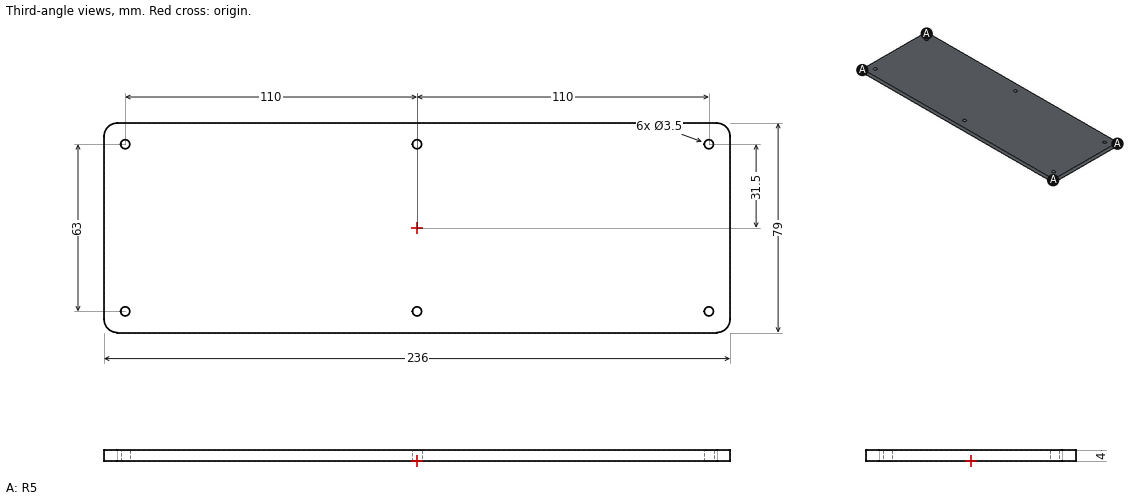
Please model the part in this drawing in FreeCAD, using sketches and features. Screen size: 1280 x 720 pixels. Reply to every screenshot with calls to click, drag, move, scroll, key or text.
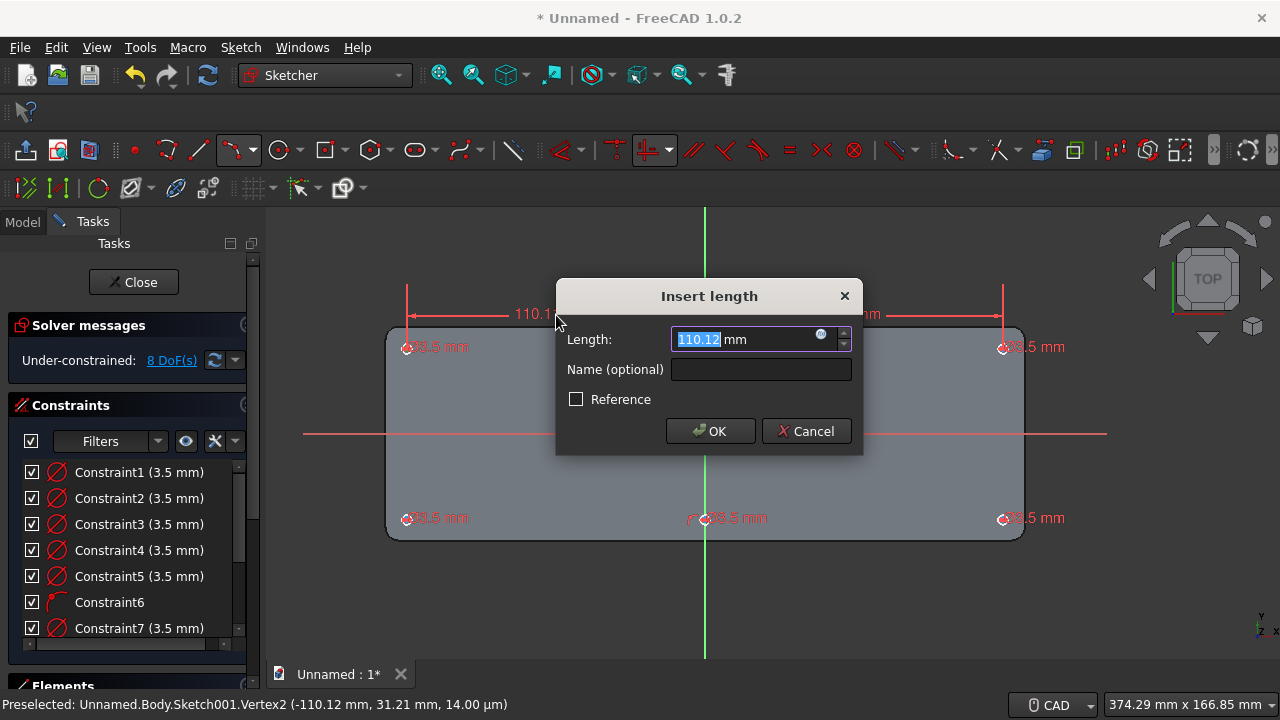
text(110)
key(Return)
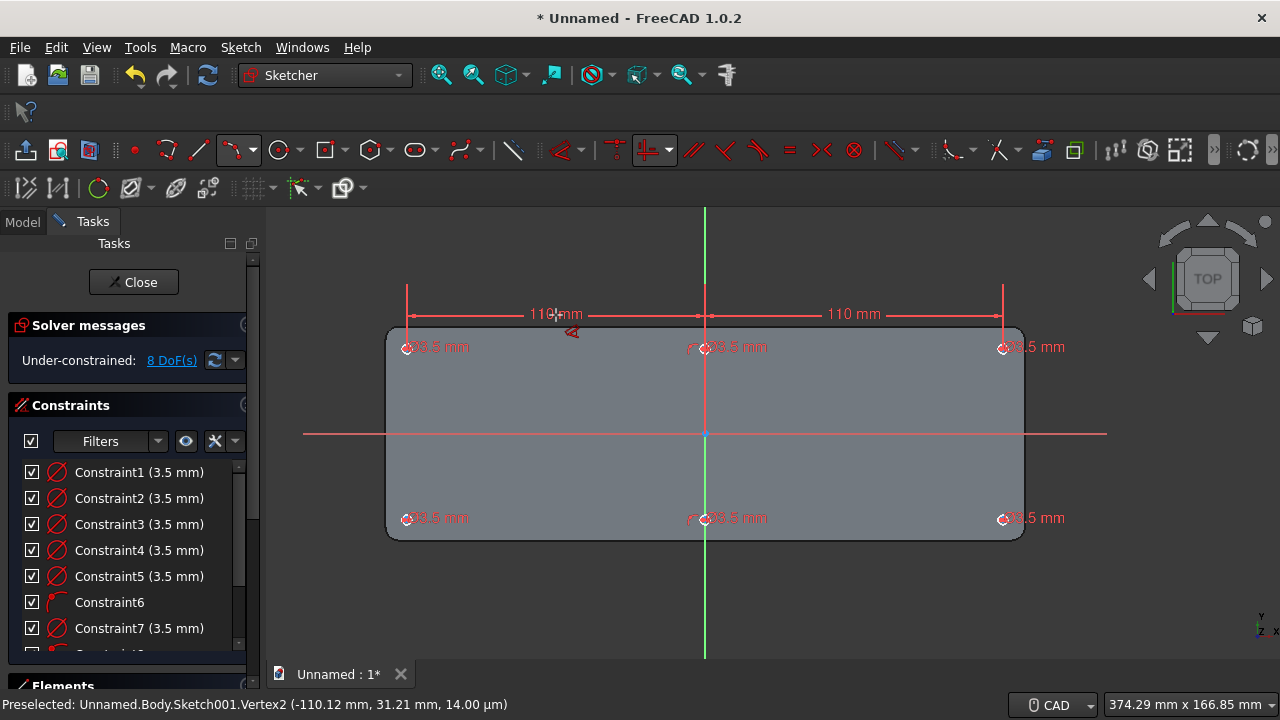
click(407, 520)
click(556, 554)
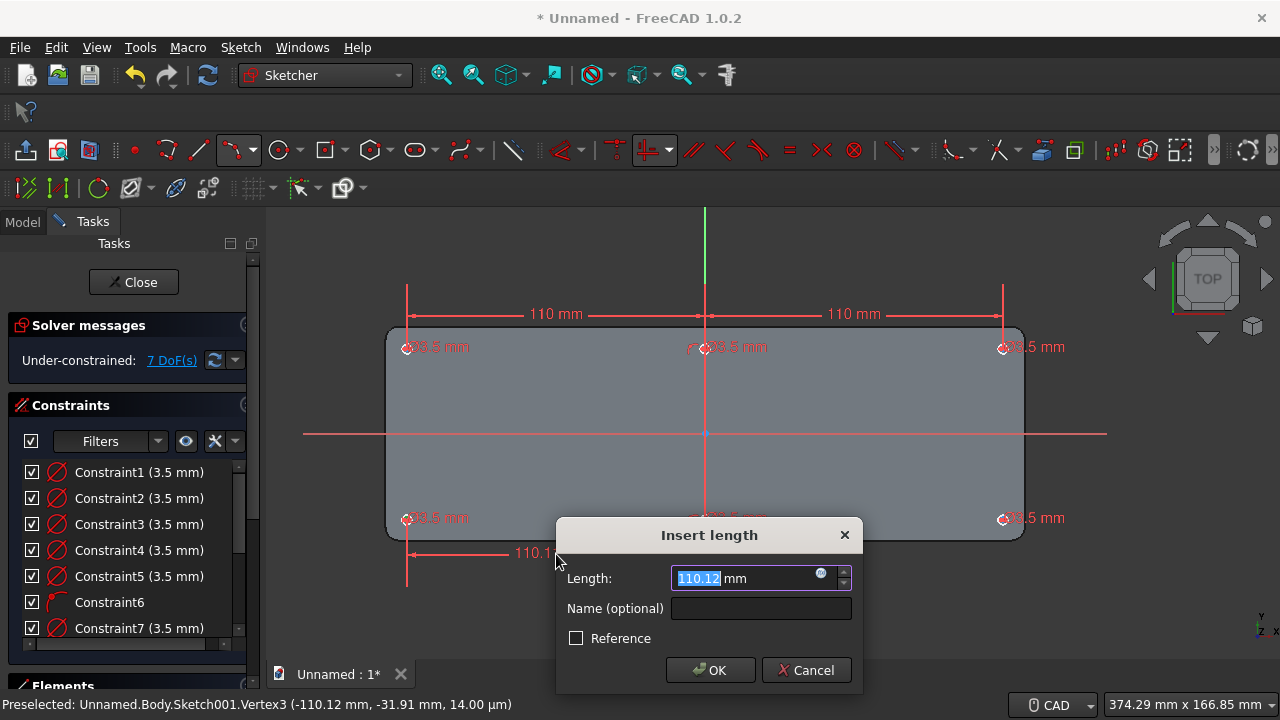
text(110)
key(Return)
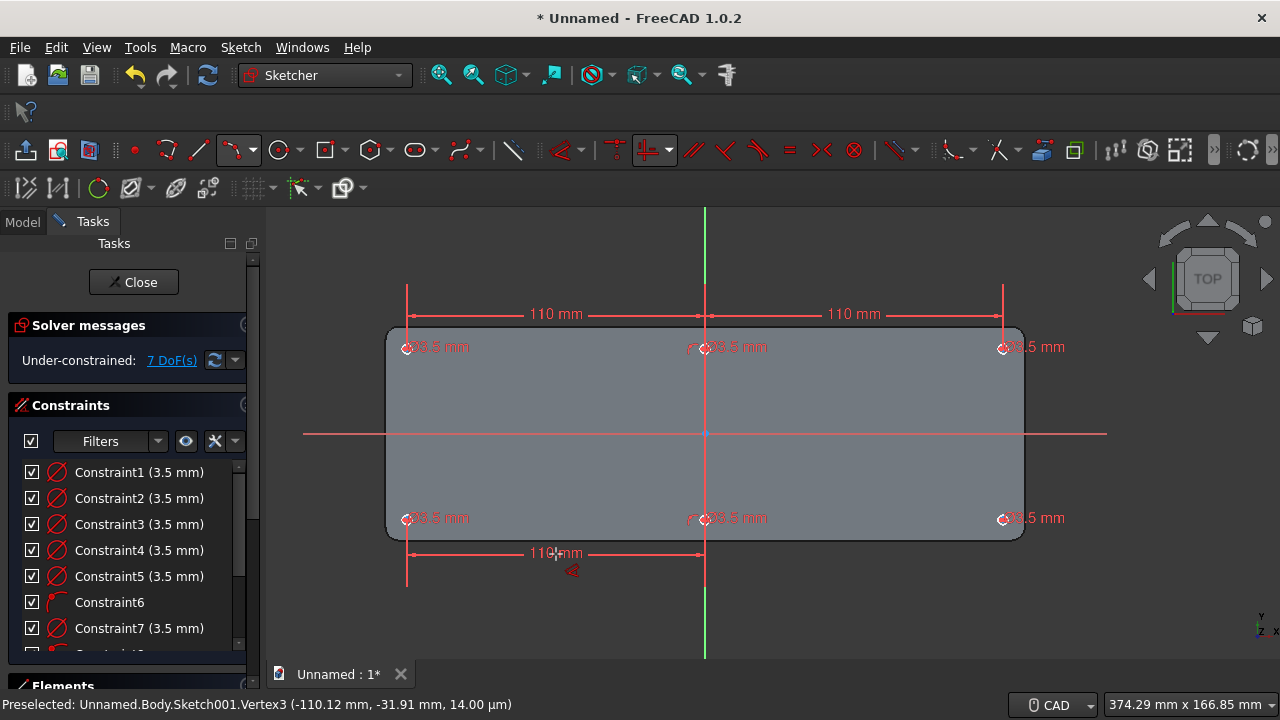
click(1003, 520)
click(854, 554)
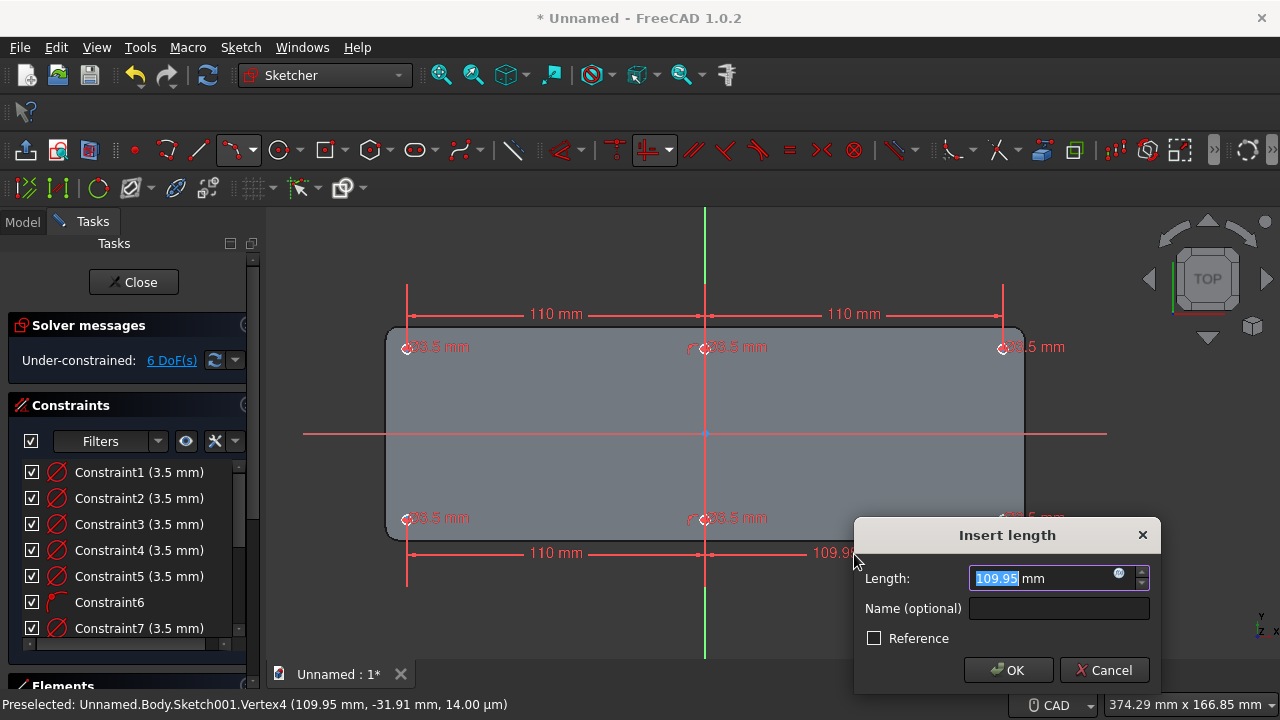
text(110)
key(Return)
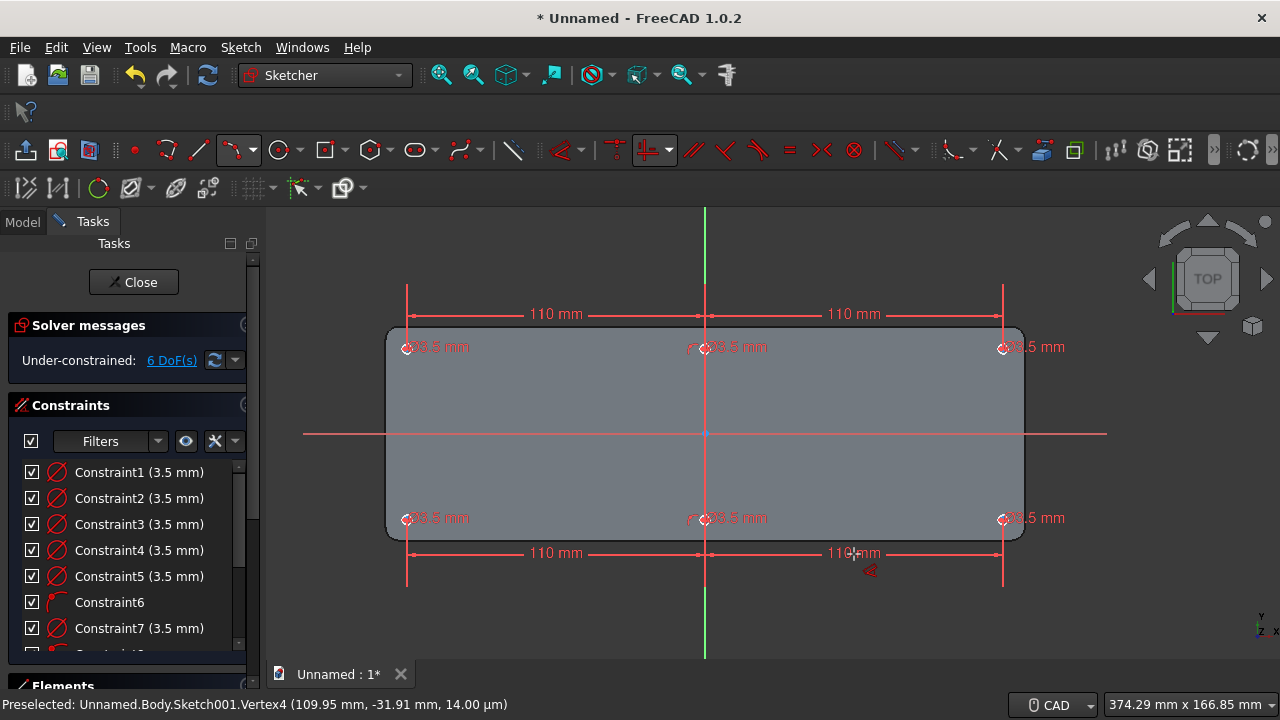
click(407, 349)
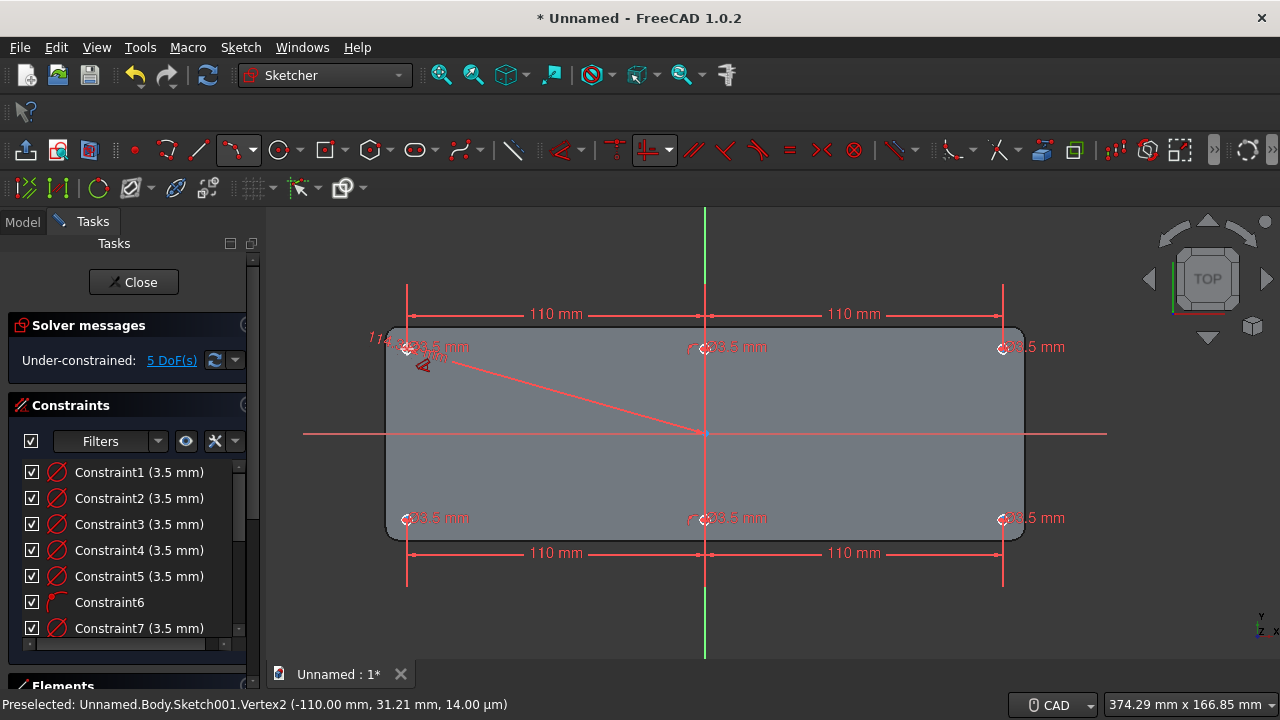
click(407, 520)
click(373, 395)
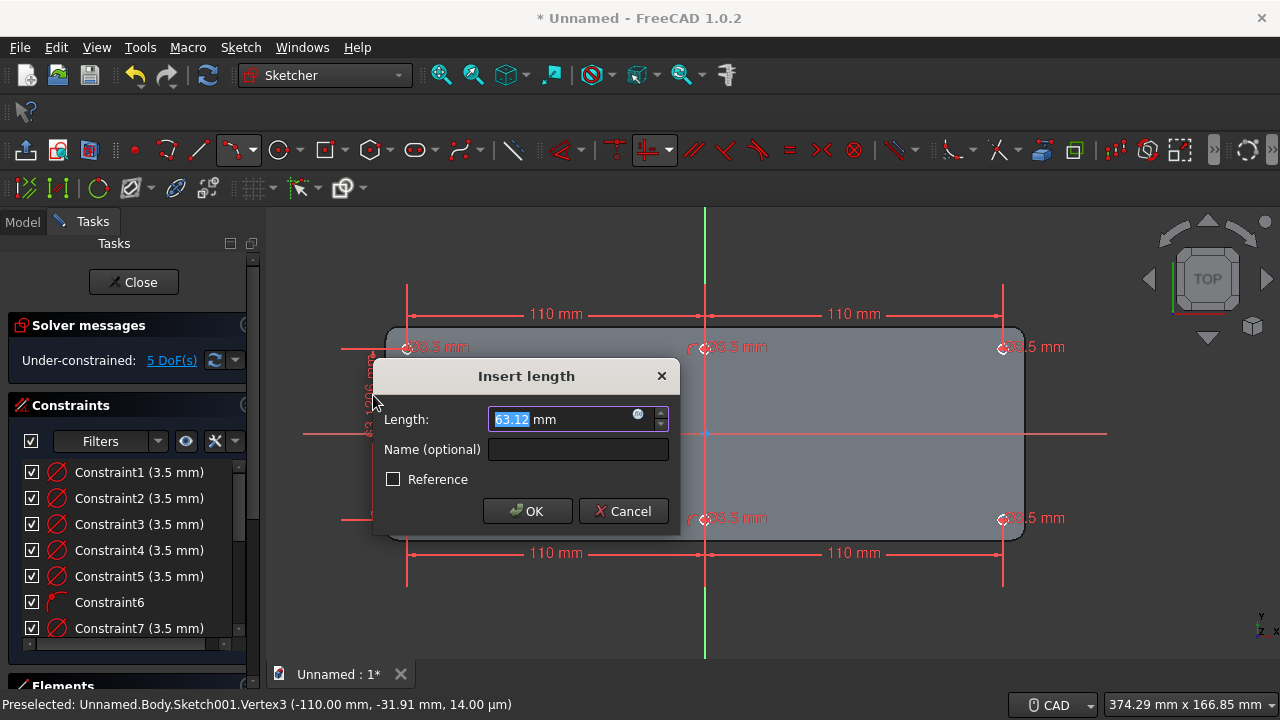
text(63)
key(Return)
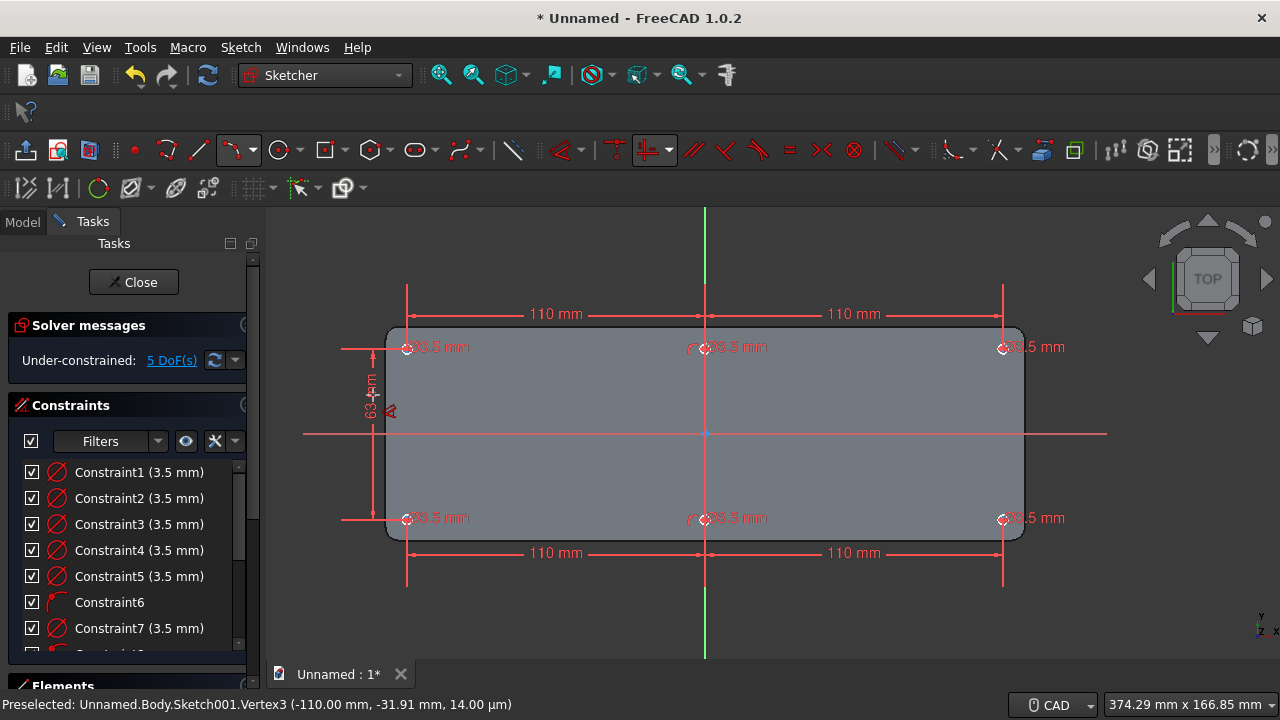
click(1003, 349)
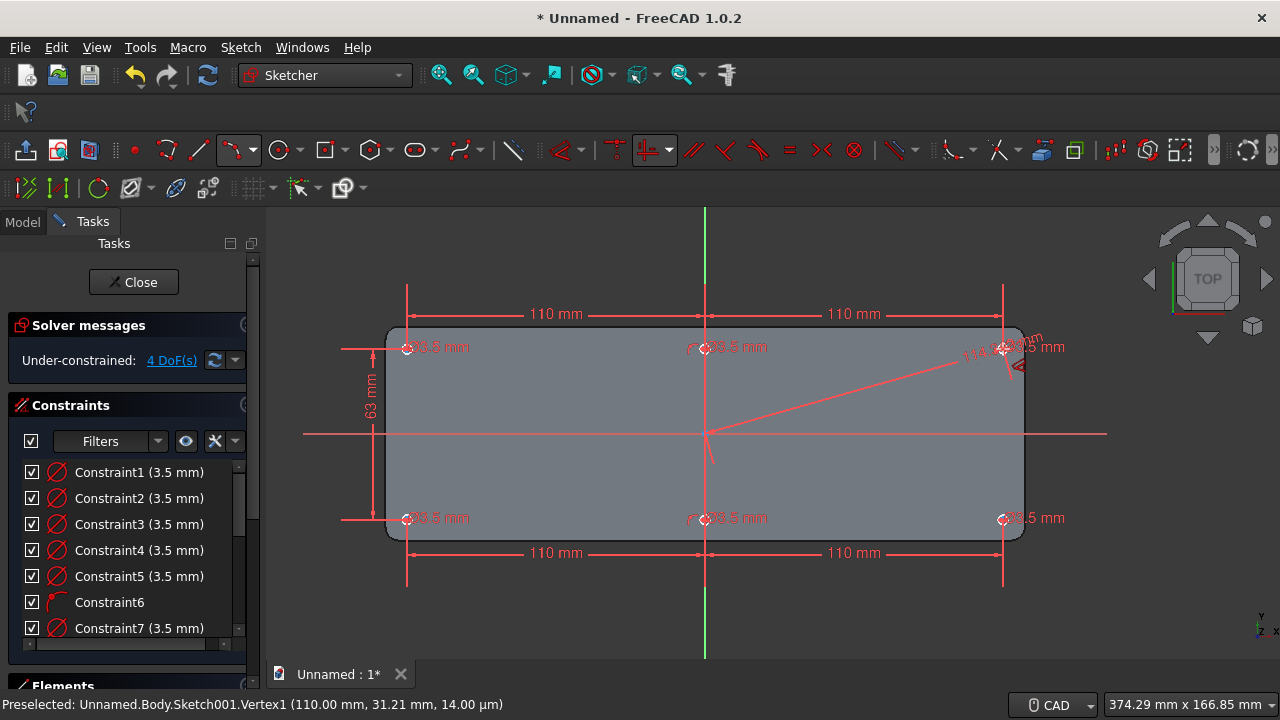
click(407, 520)
click(1037, 395)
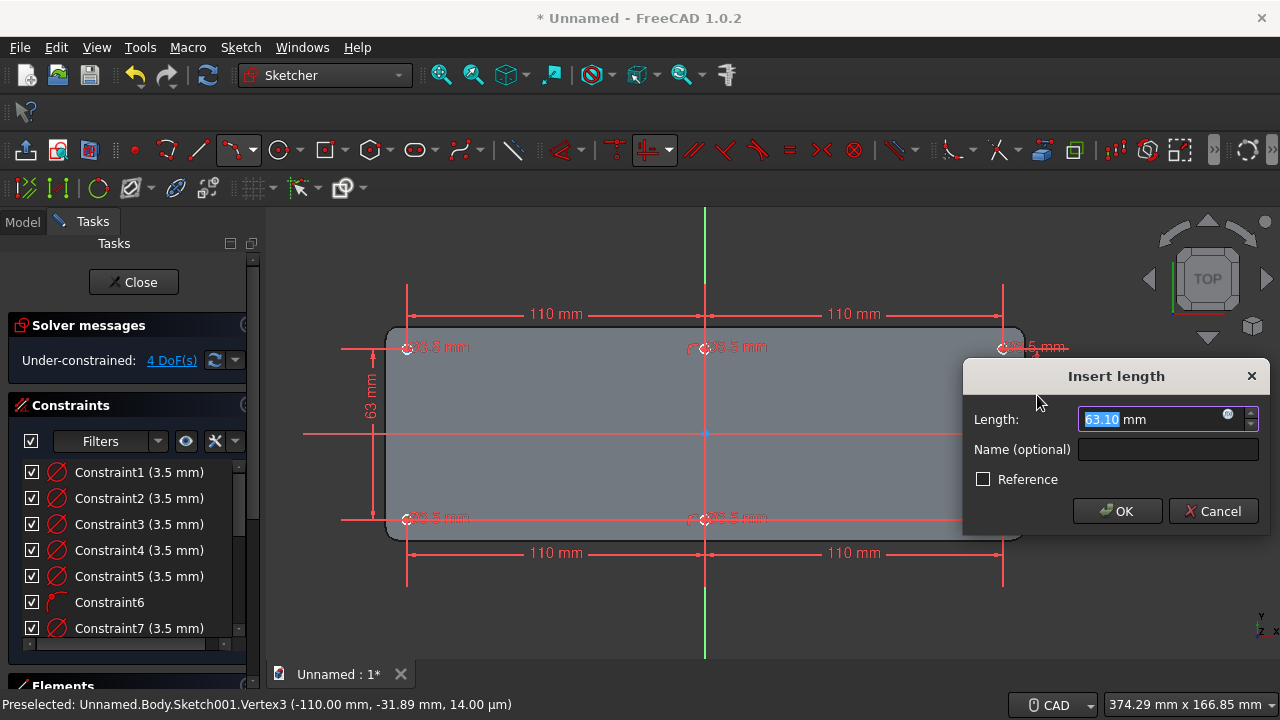
text(63)
key(Return)